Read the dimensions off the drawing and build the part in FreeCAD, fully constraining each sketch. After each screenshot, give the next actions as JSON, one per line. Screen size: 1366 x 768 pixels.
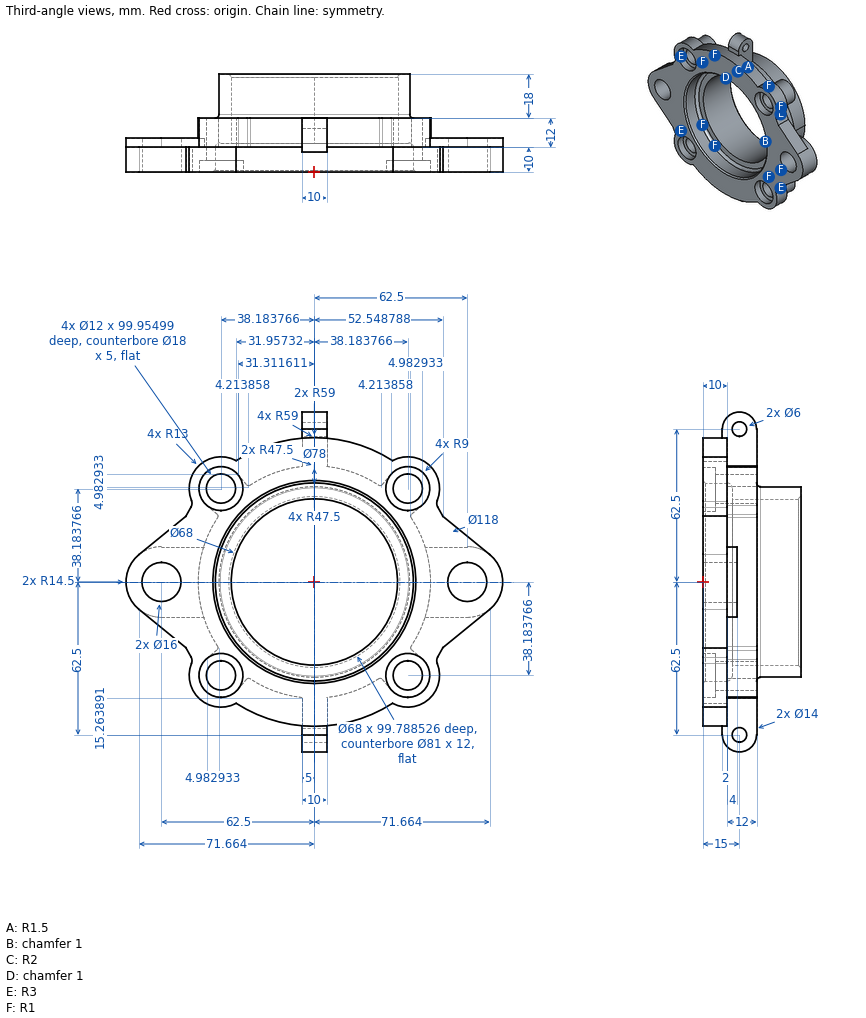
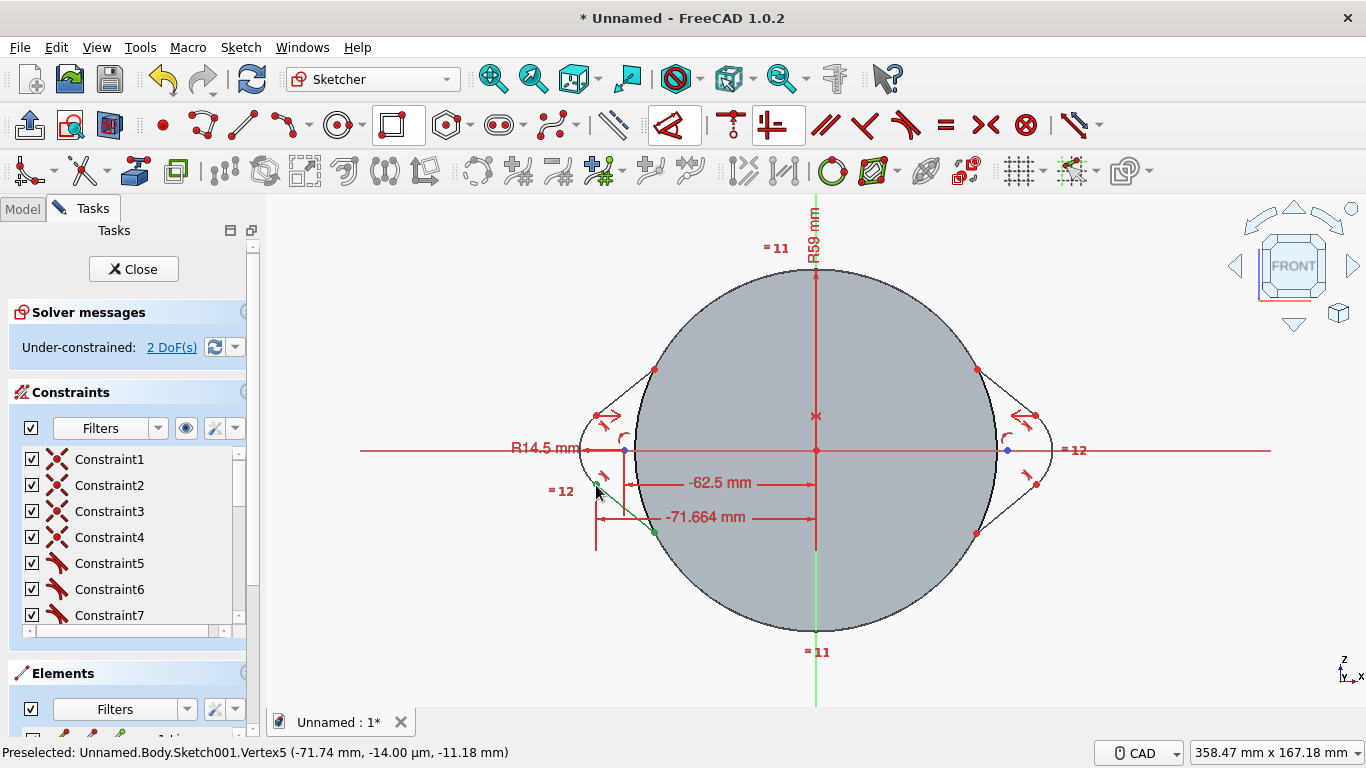
{"action": "left_click", "coordinate": [1036, 485]}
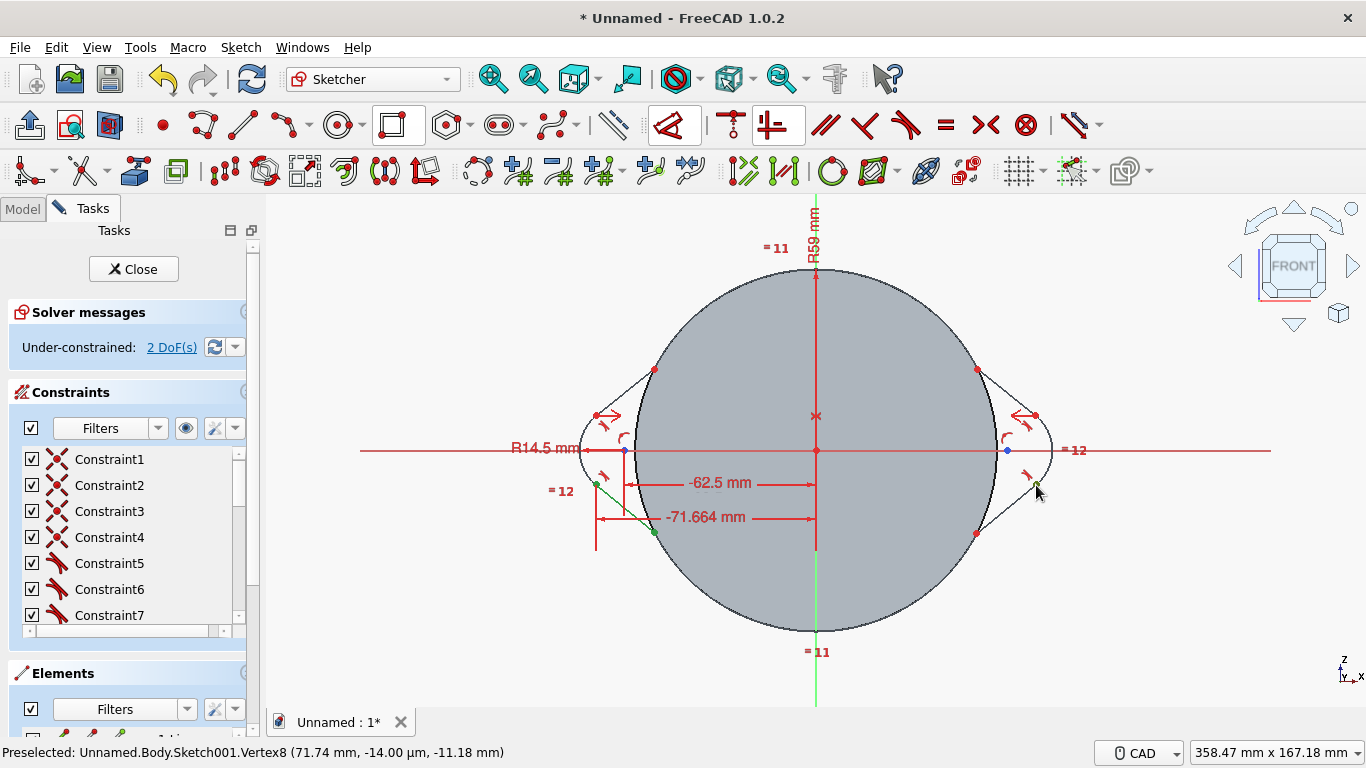
{"action": "left_click", "coordinate": [696, 126]}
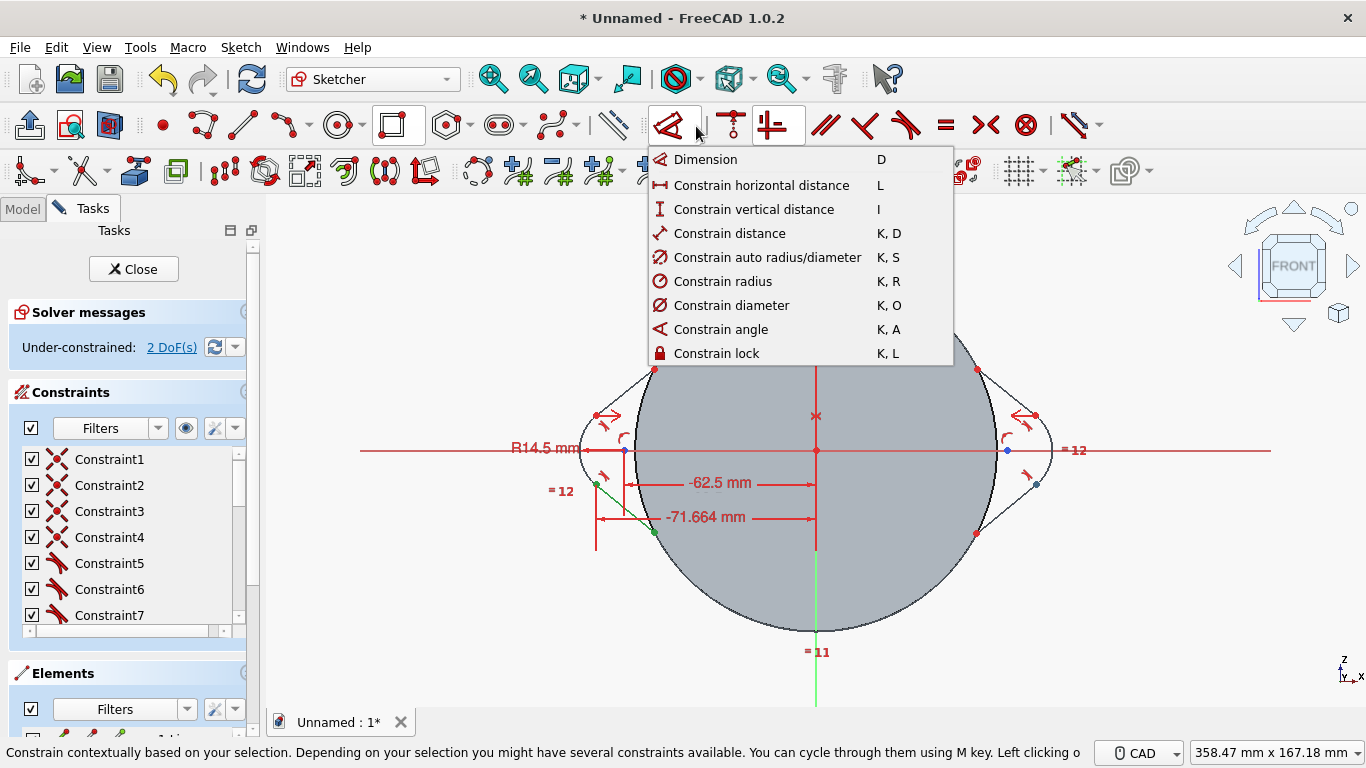
{"action": "left_click", "coordinate": [801, 185]}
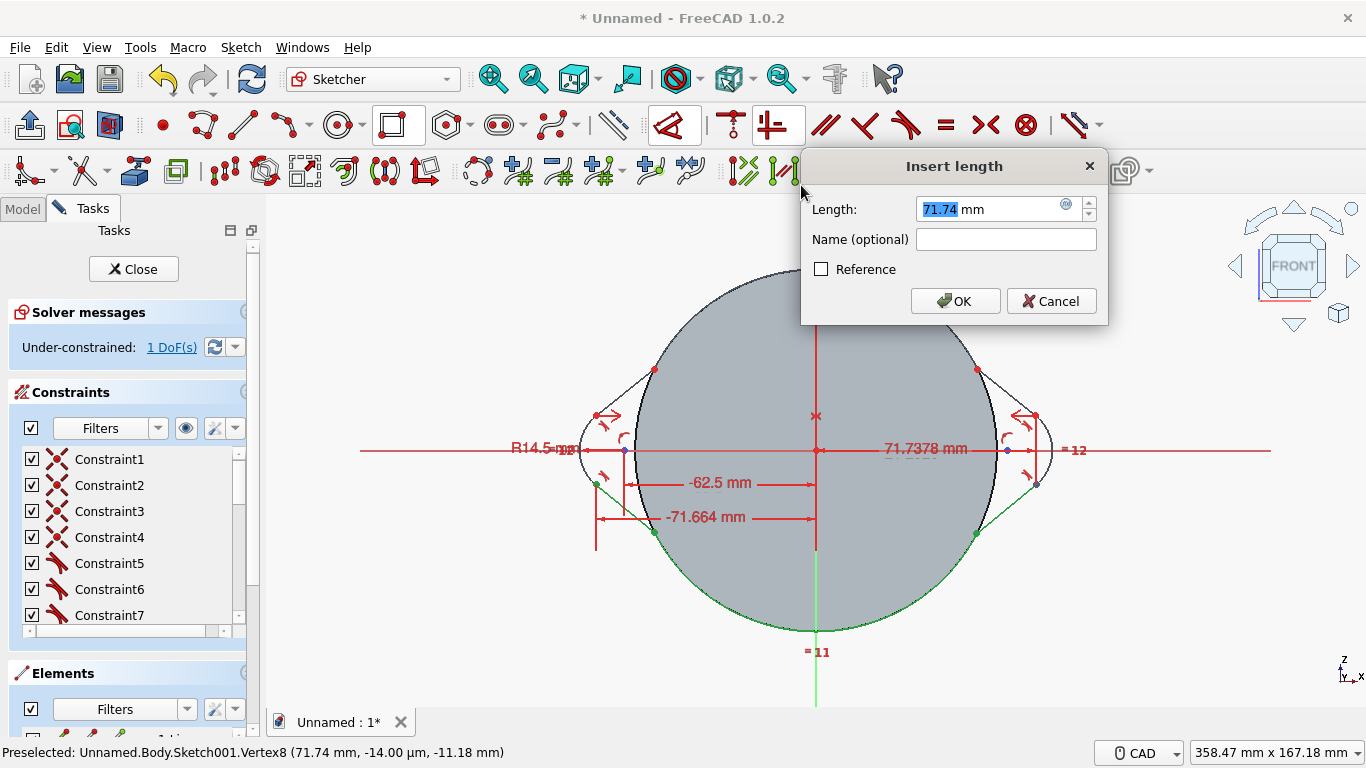
{"action": "type", "text": "71.664"}
{"action": "key", "text": "Return"}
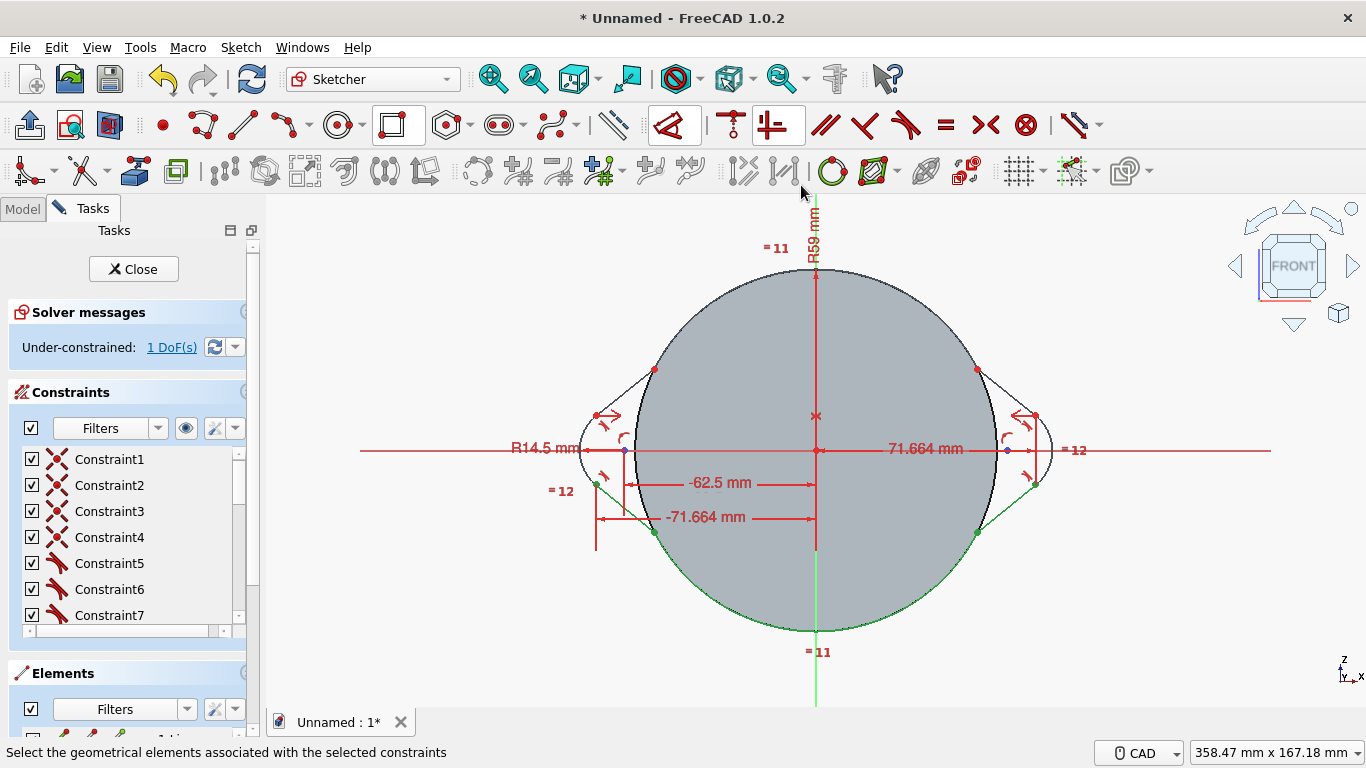
{"action": "left_click", "coordinate": [978, 369]}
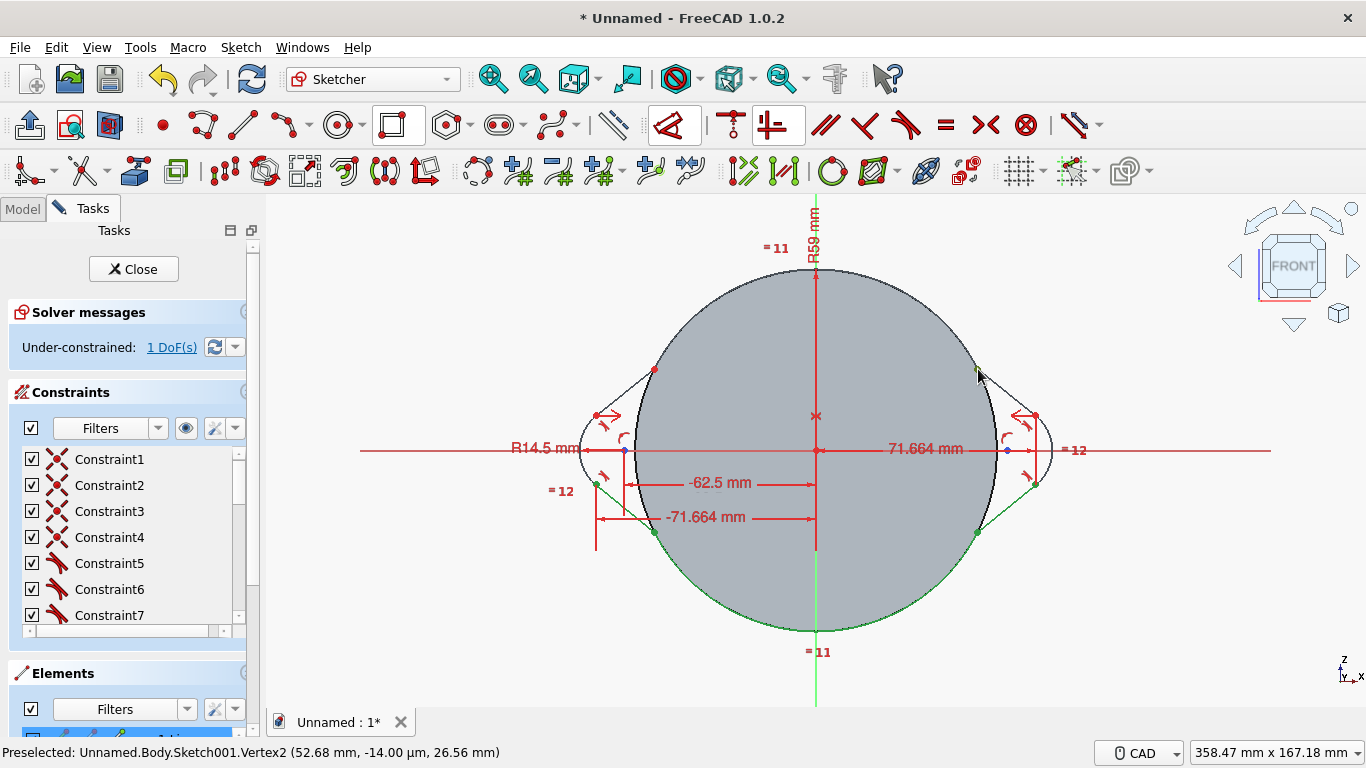
{"action": "key", "text": "l"}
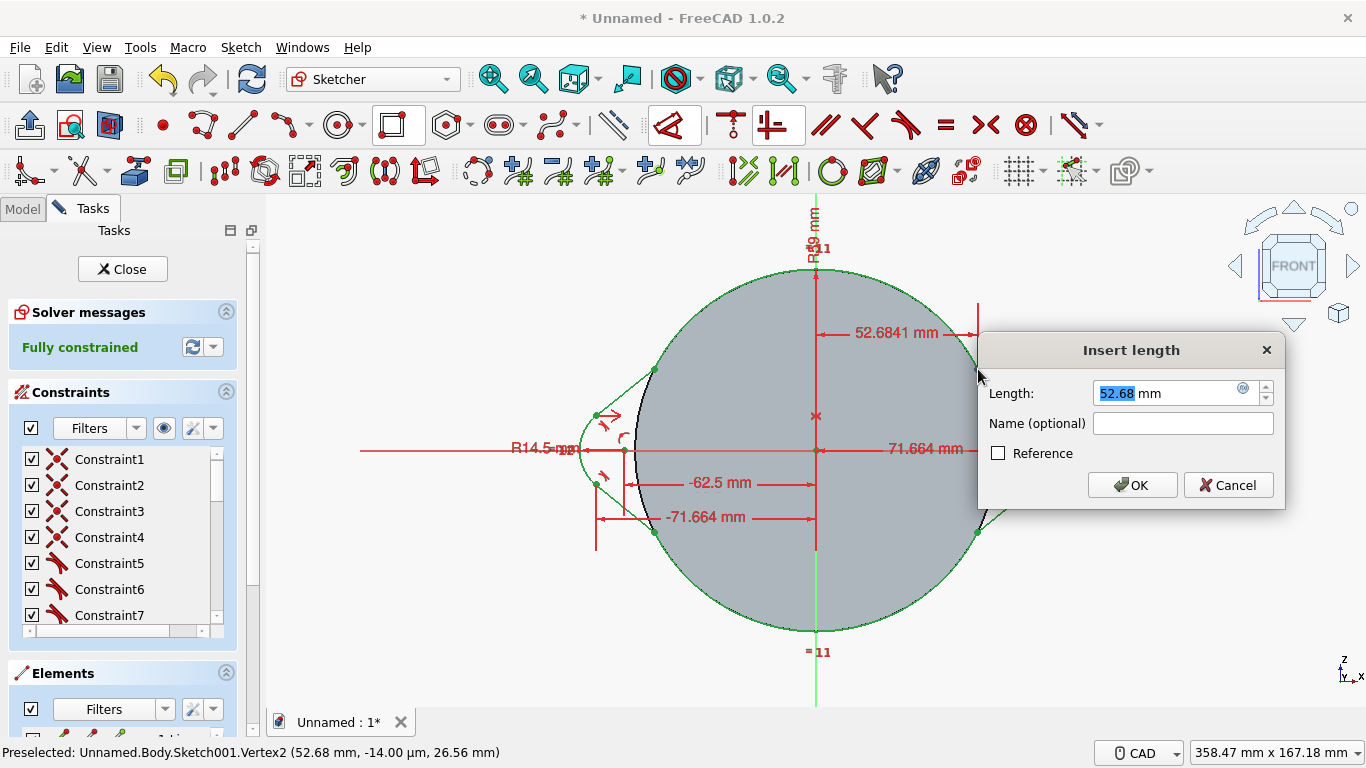
{"action": "type", "text": "52.548788"}
{"action": "key", "text": "Return"}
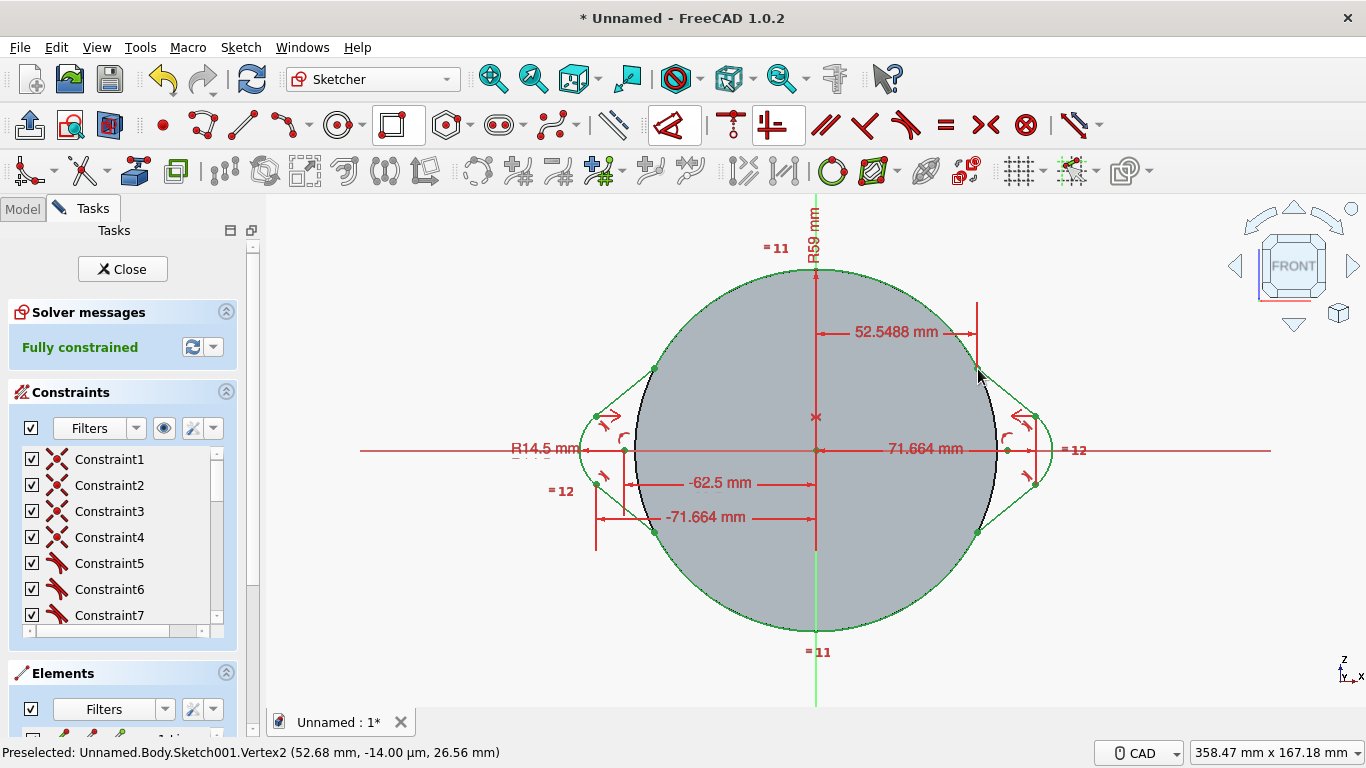
{"action": "left_click", "coordinate": [123, 269]}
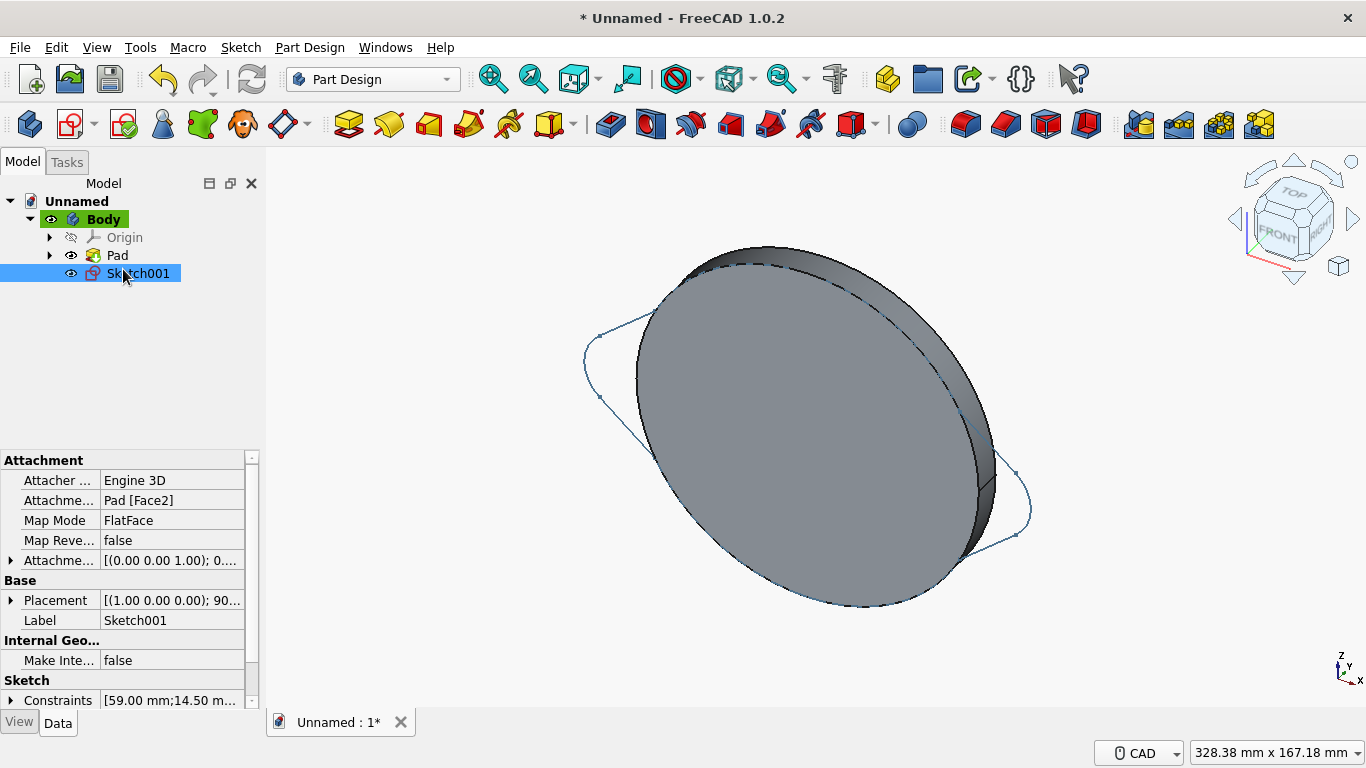
{"action": "left_click", "coordinate": [350, 124]}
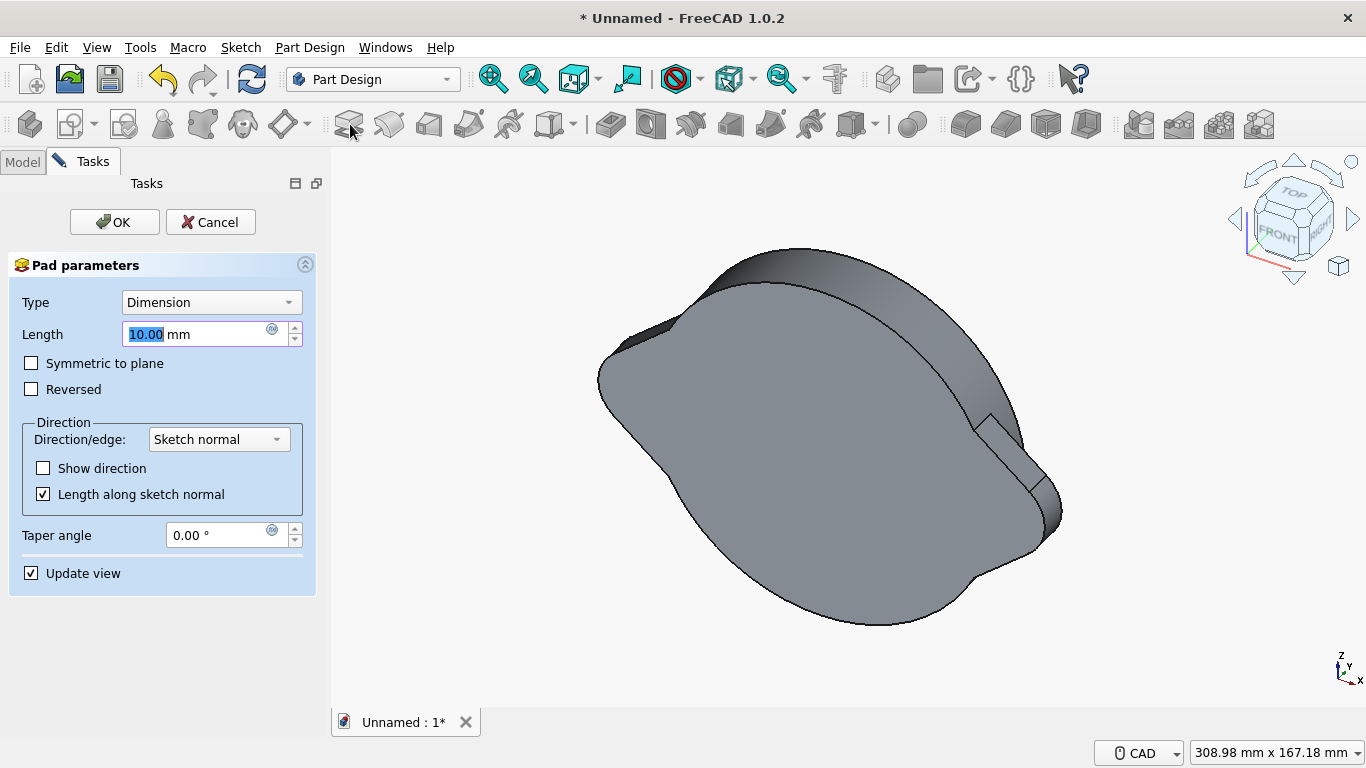
{"action": "type", "text": "10"}
{"action": "key", "text": "Tab"}